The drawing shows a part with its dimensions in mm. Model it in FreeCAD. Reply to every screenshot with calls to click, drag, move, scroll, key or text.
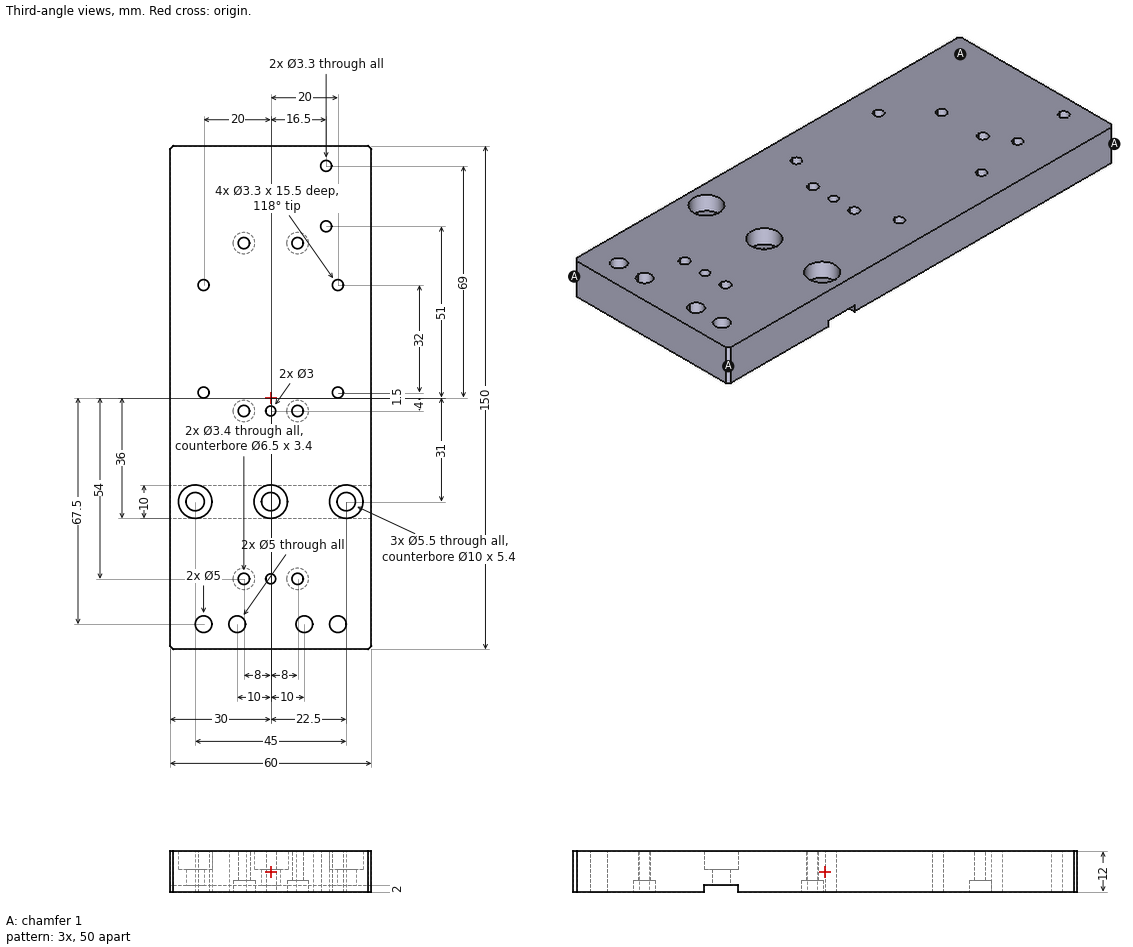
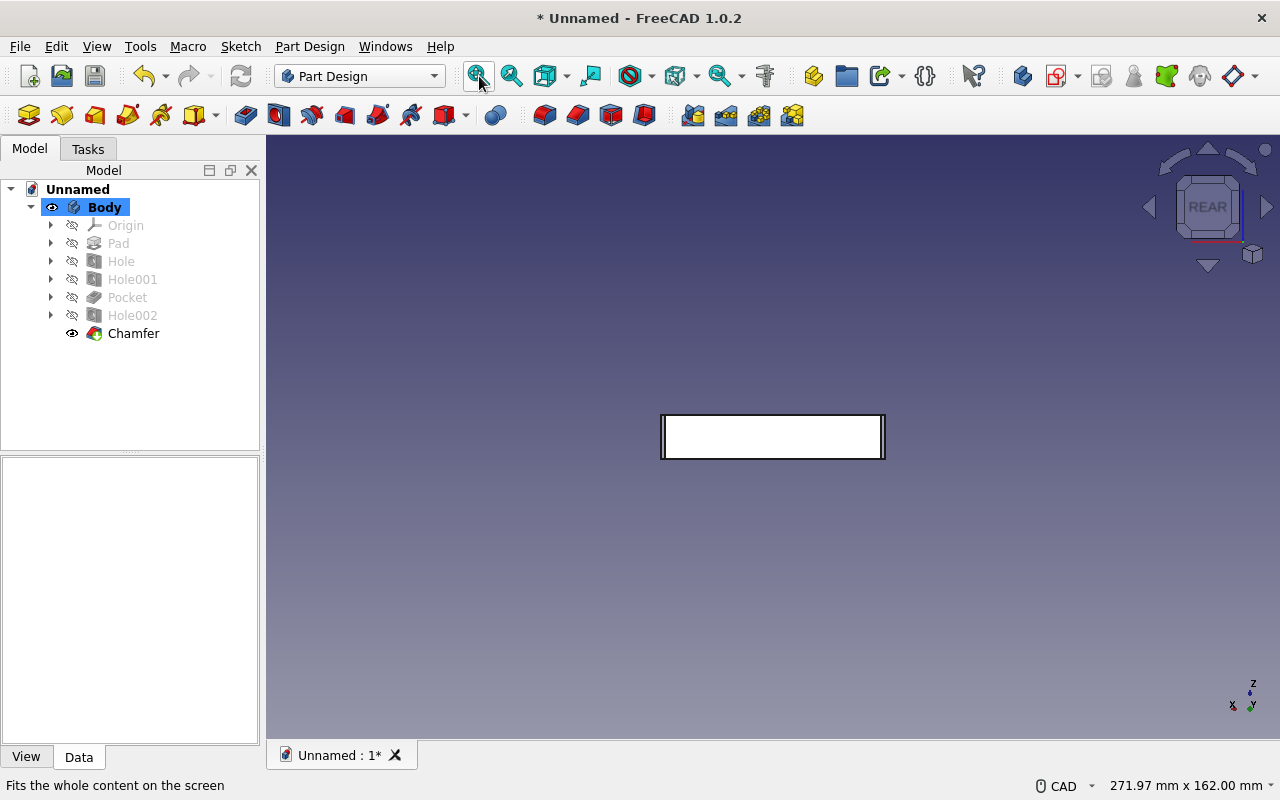
key(5)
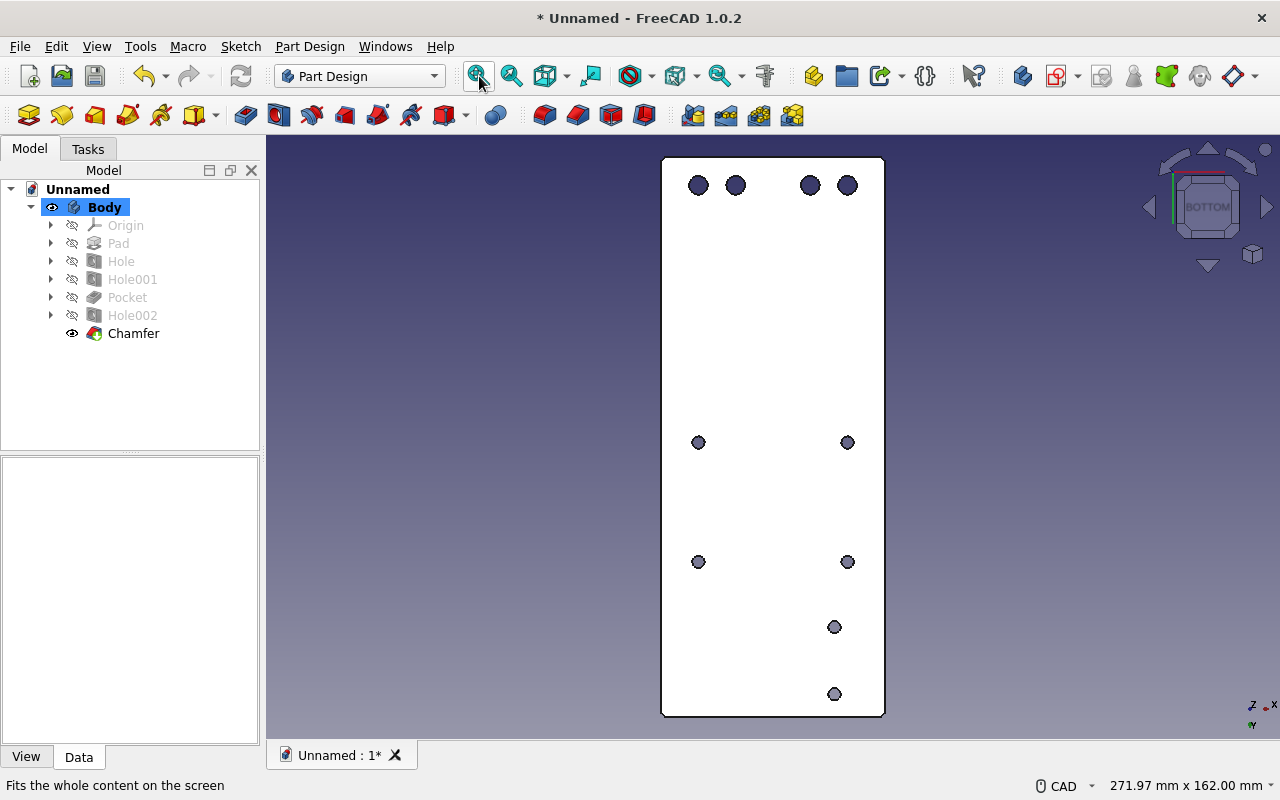
click(773, 356)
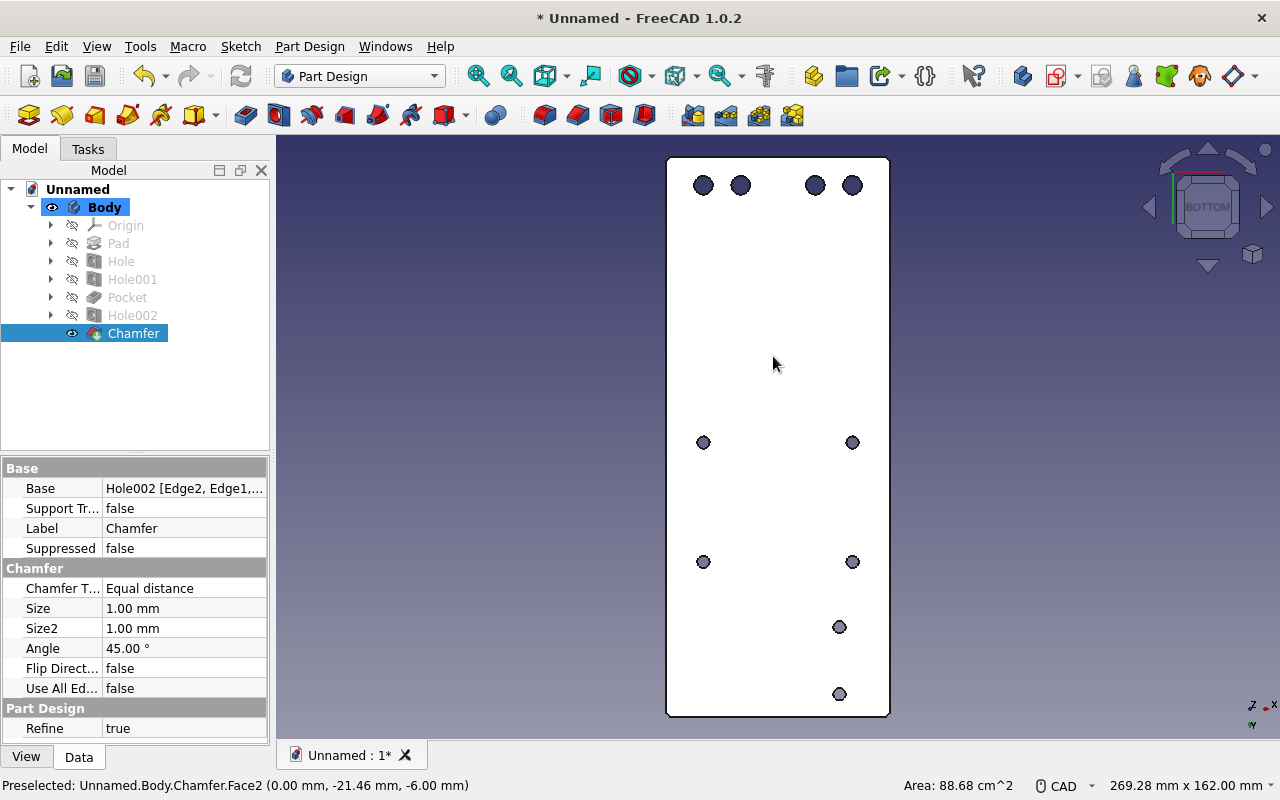
click(1056, 76)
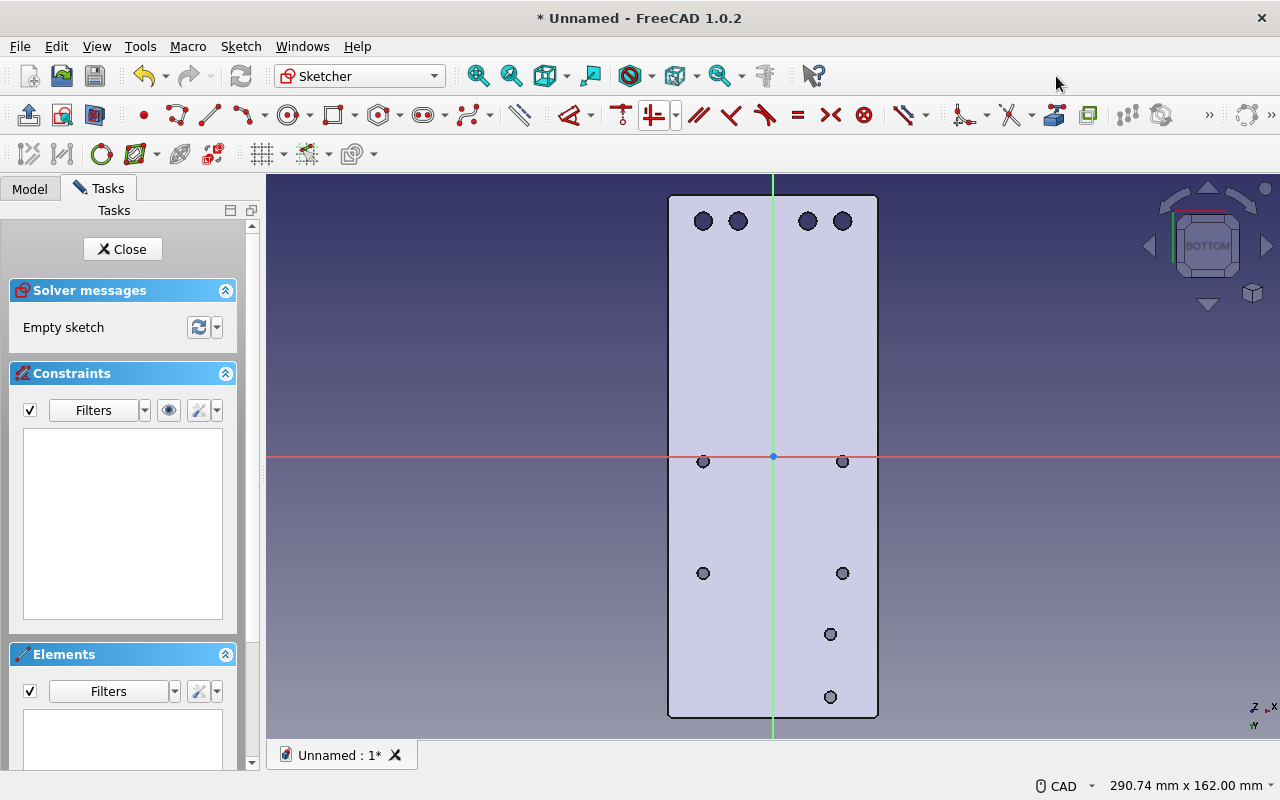
scroll(782, 245, up, 11)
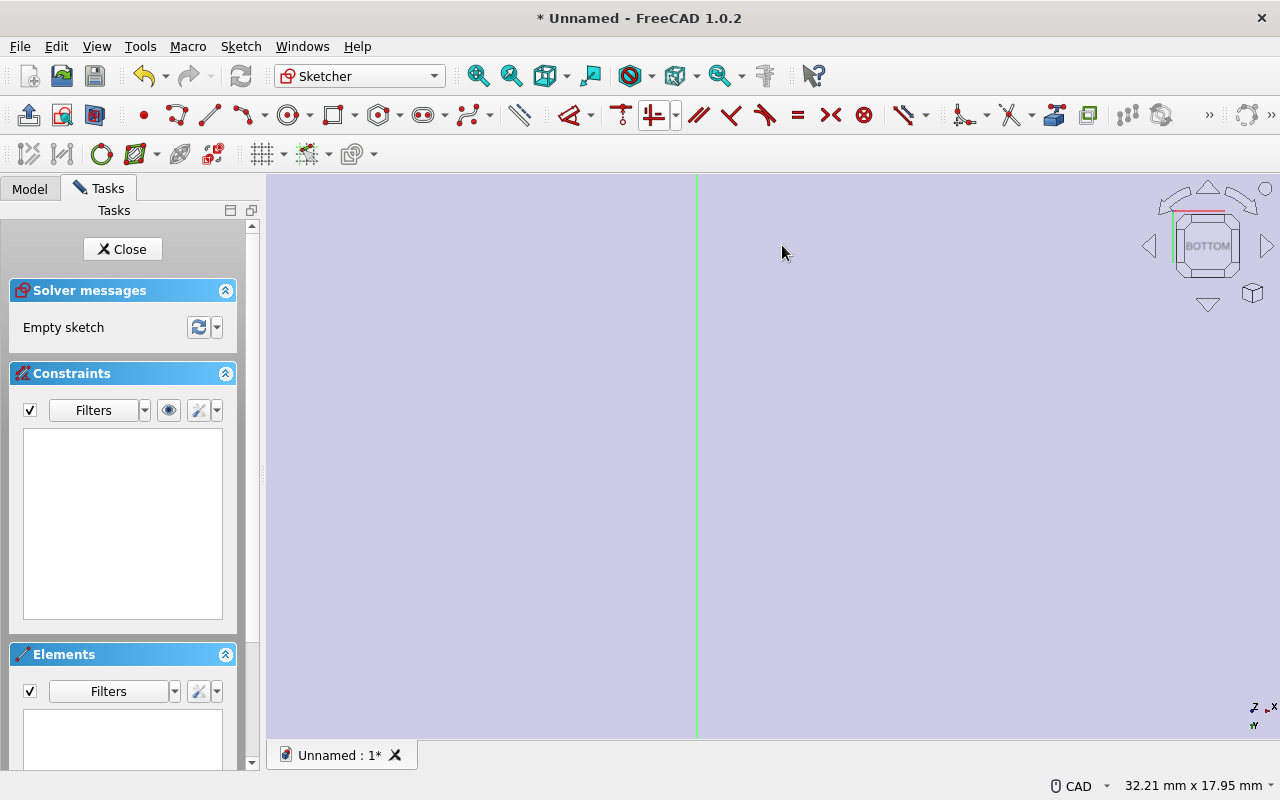
click(288, 116)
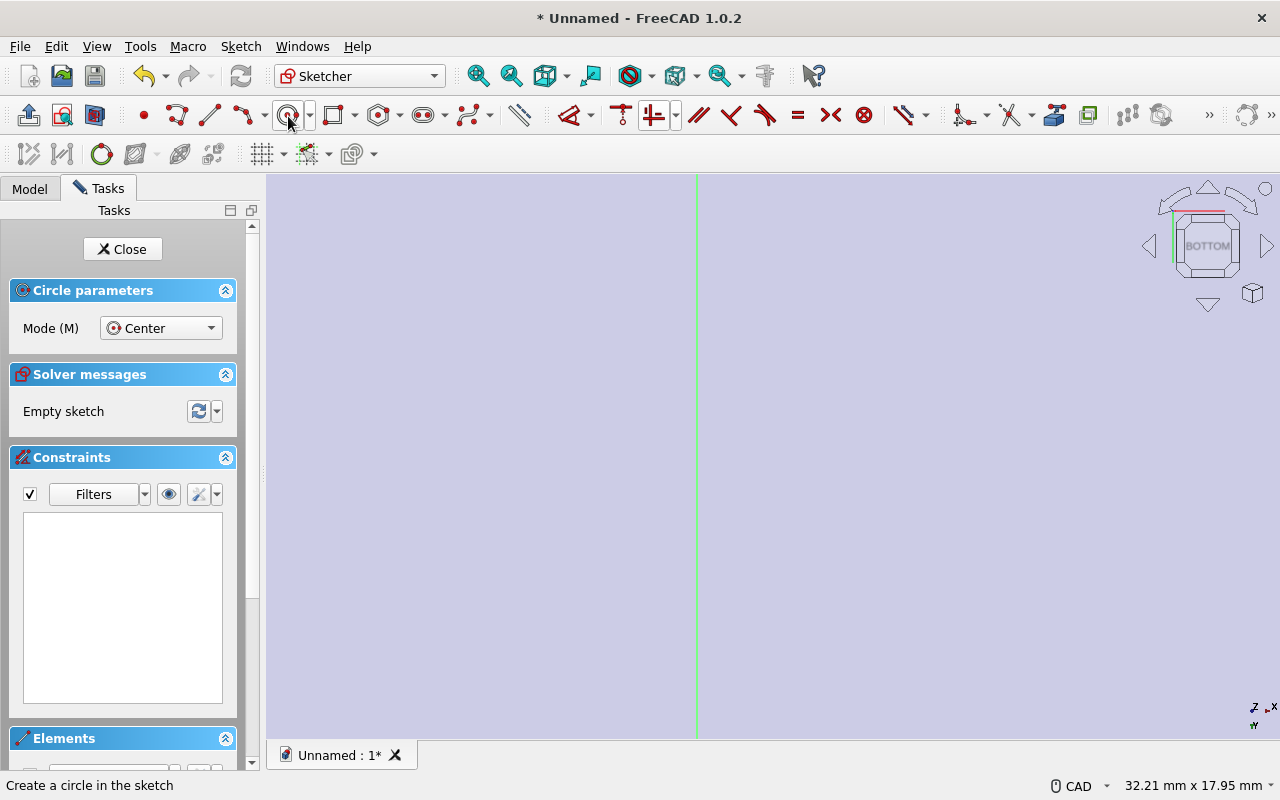
click(445, 453)
click(483, 415)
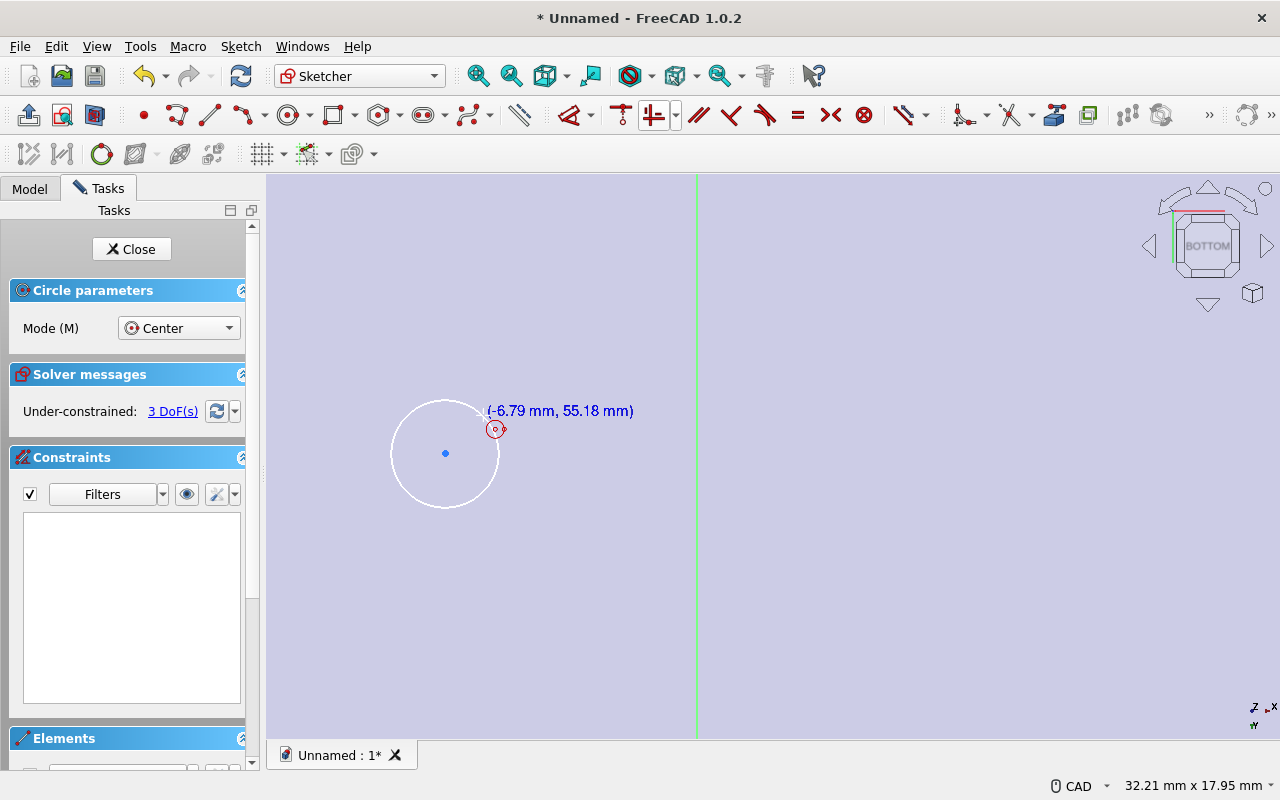
click(948, 453)
click(986, 415)
key(Escape)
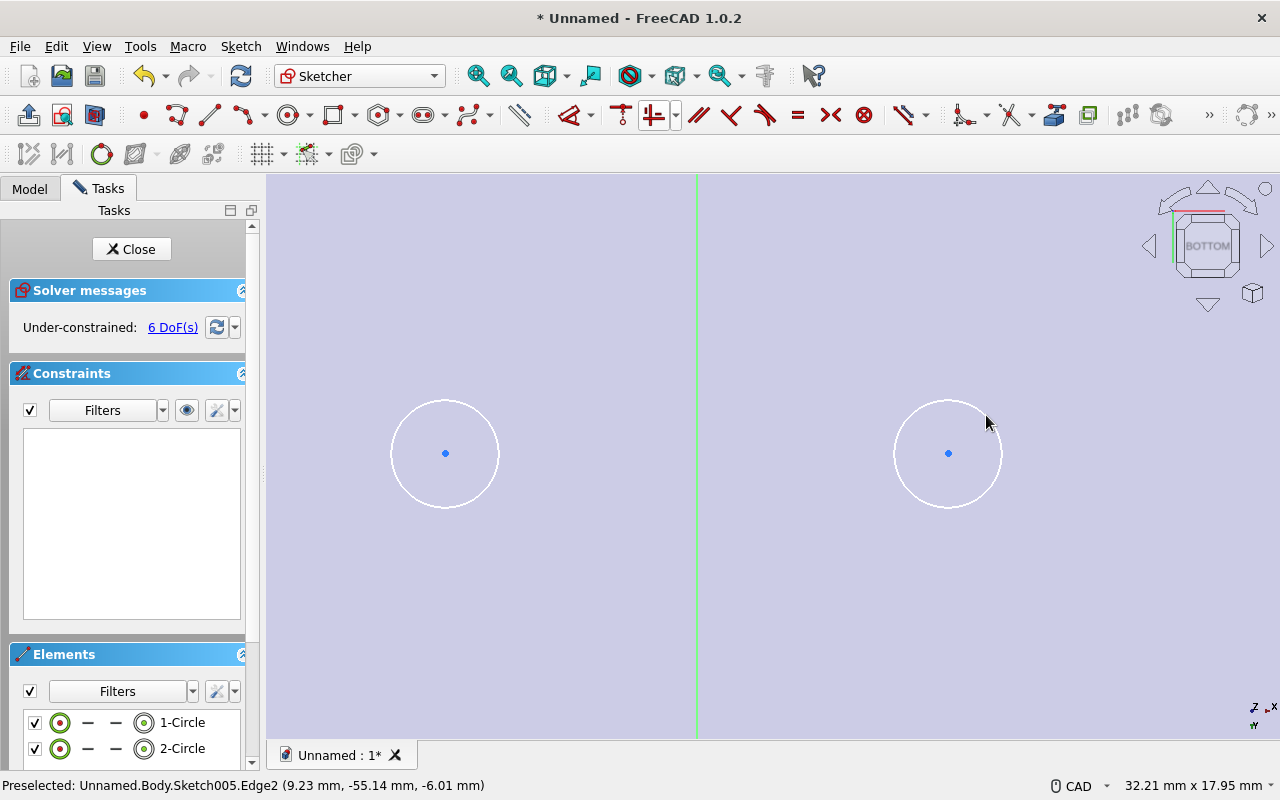
click(483, 416)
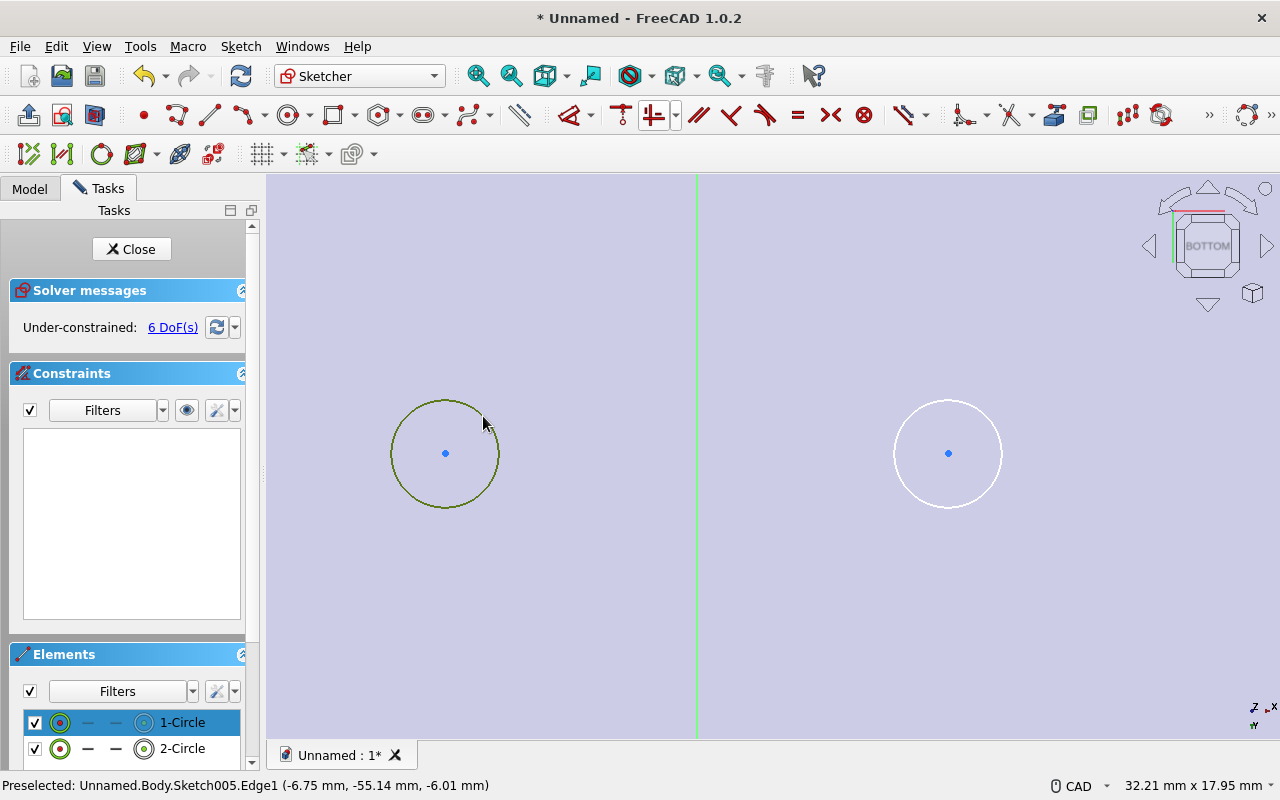
click(986, 416)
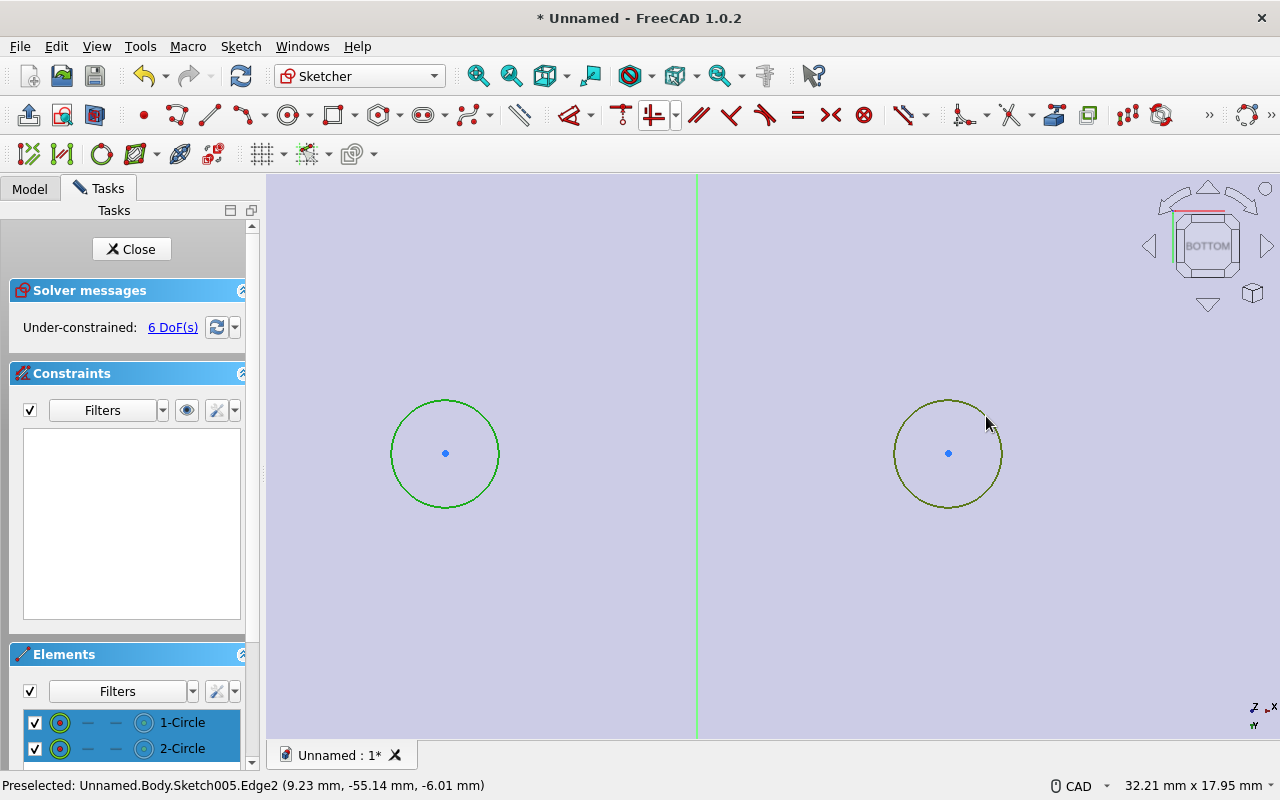
click(798, 116)